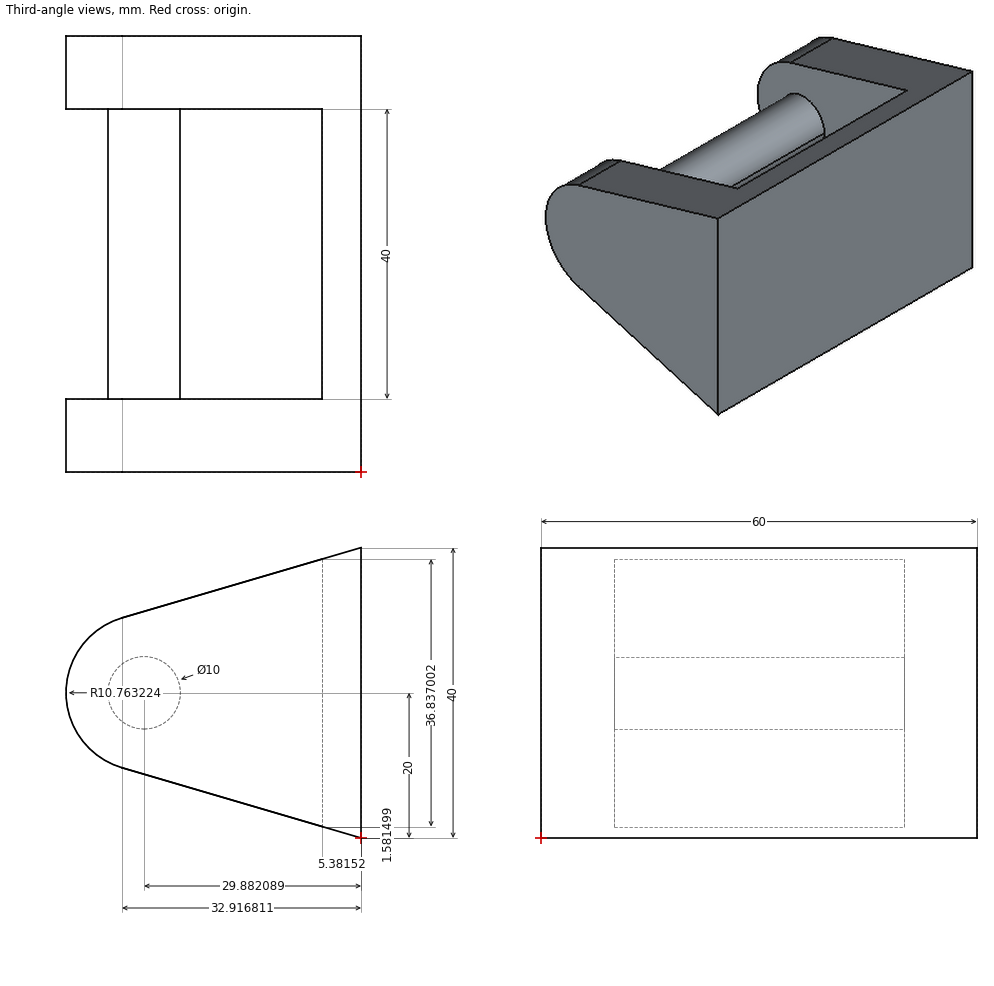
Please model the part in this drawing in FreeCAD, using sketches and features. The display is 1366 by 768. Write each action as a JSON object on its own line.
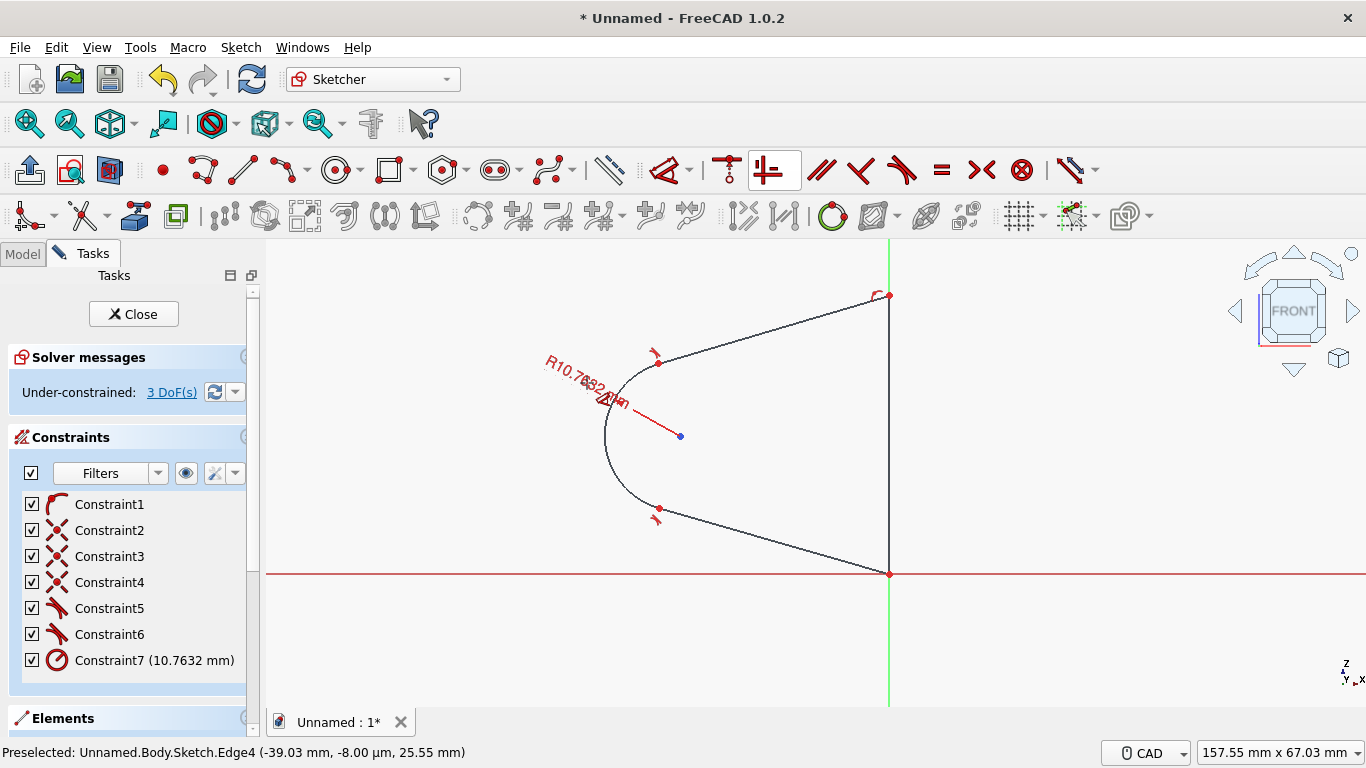
{"action": "left_click", "coordinate": [889, 379]}
{"action": "left_click", "coordinate": [923, 435]}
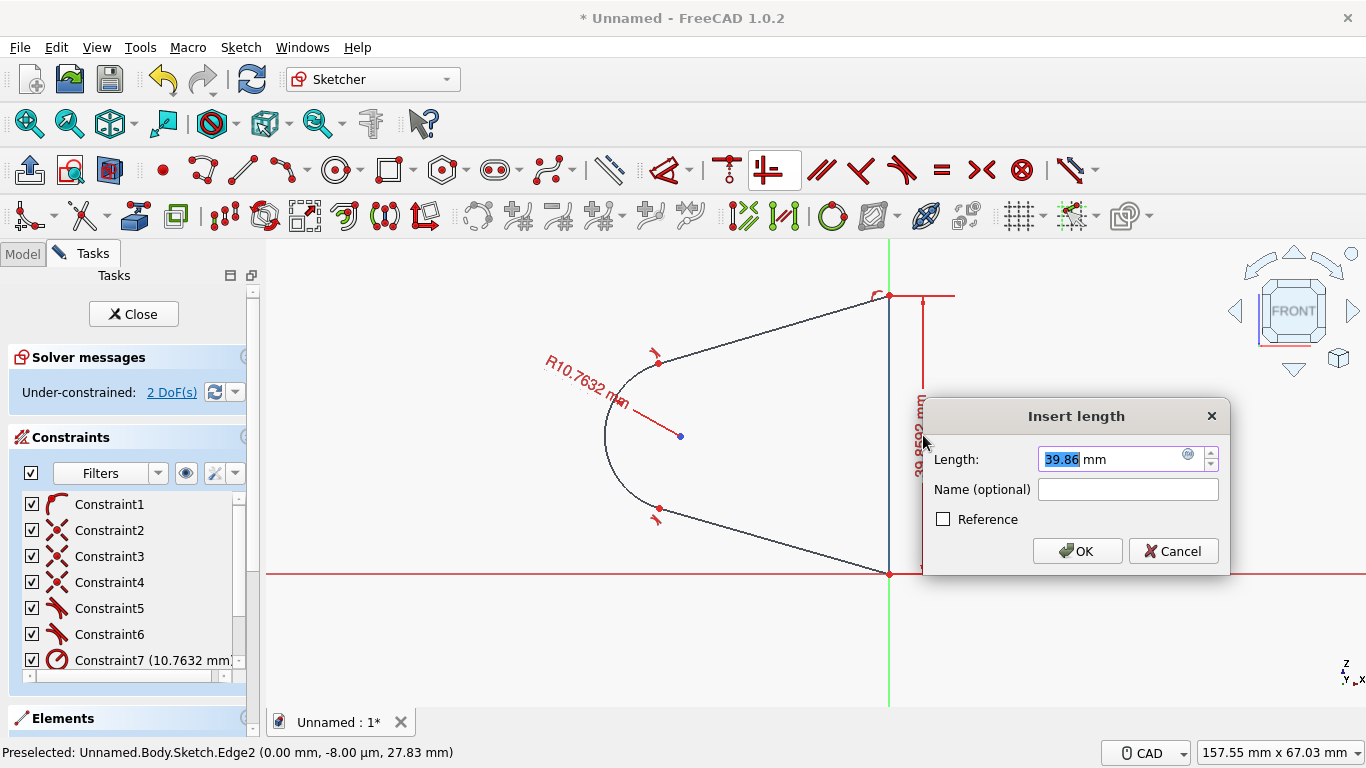
{"action": "type", "text": "40"}
{"action": "key", "text": "Return"}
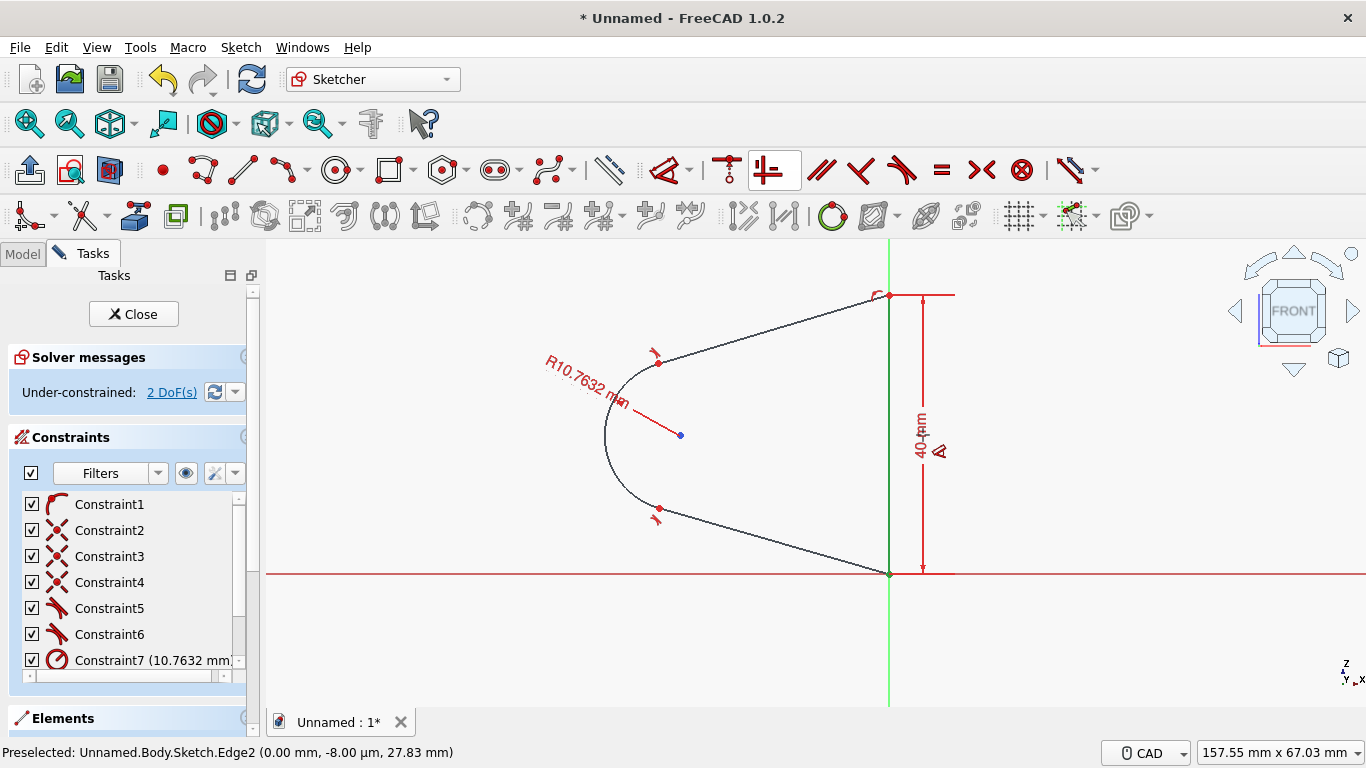
{"action": "left_click", "coordinate": [680, 436]}
{"action": "left_click", "coordinate": [923, 505]}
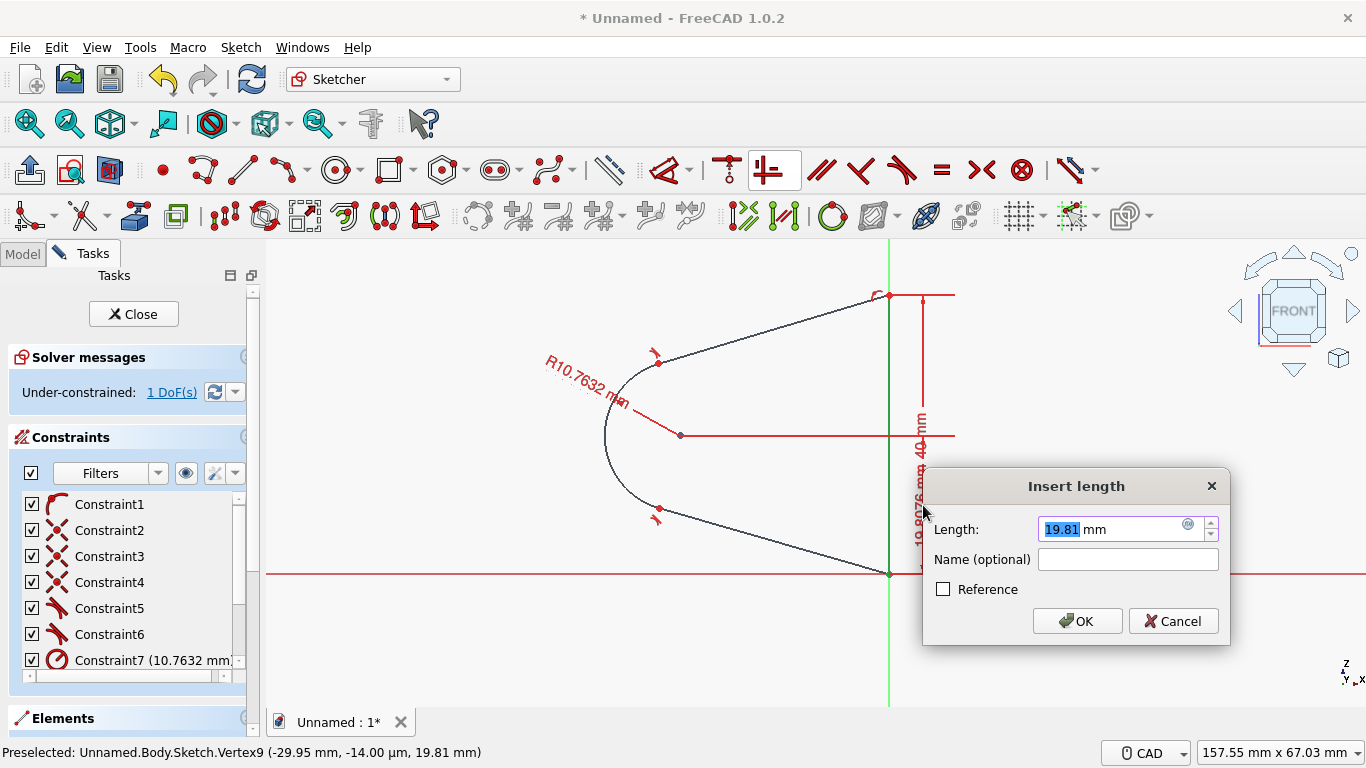
{"action": "type", "text": "20"}
{"action": "key", "text": "Return"}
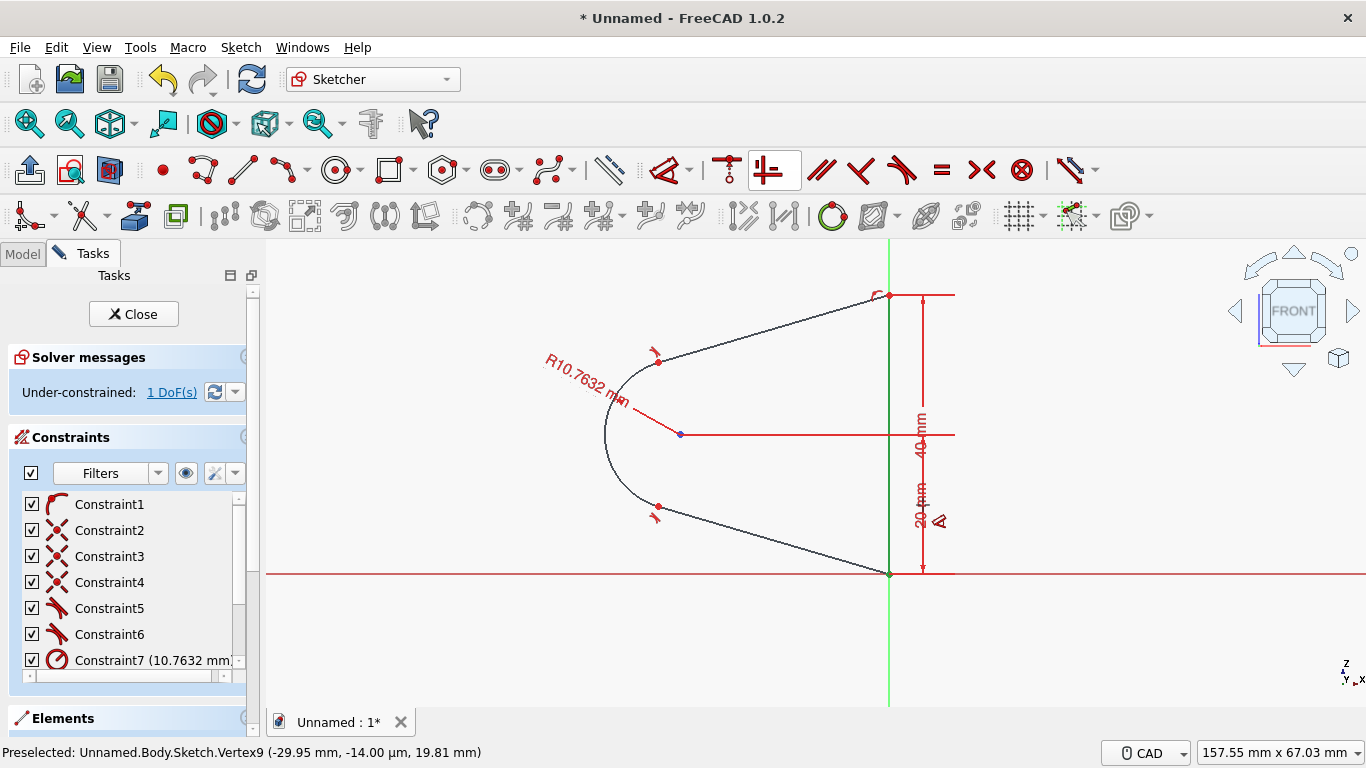
{"action": "left_click", "coordinate": [659, 363]}
{"action": "left_click", "coordinate": [774, 608]}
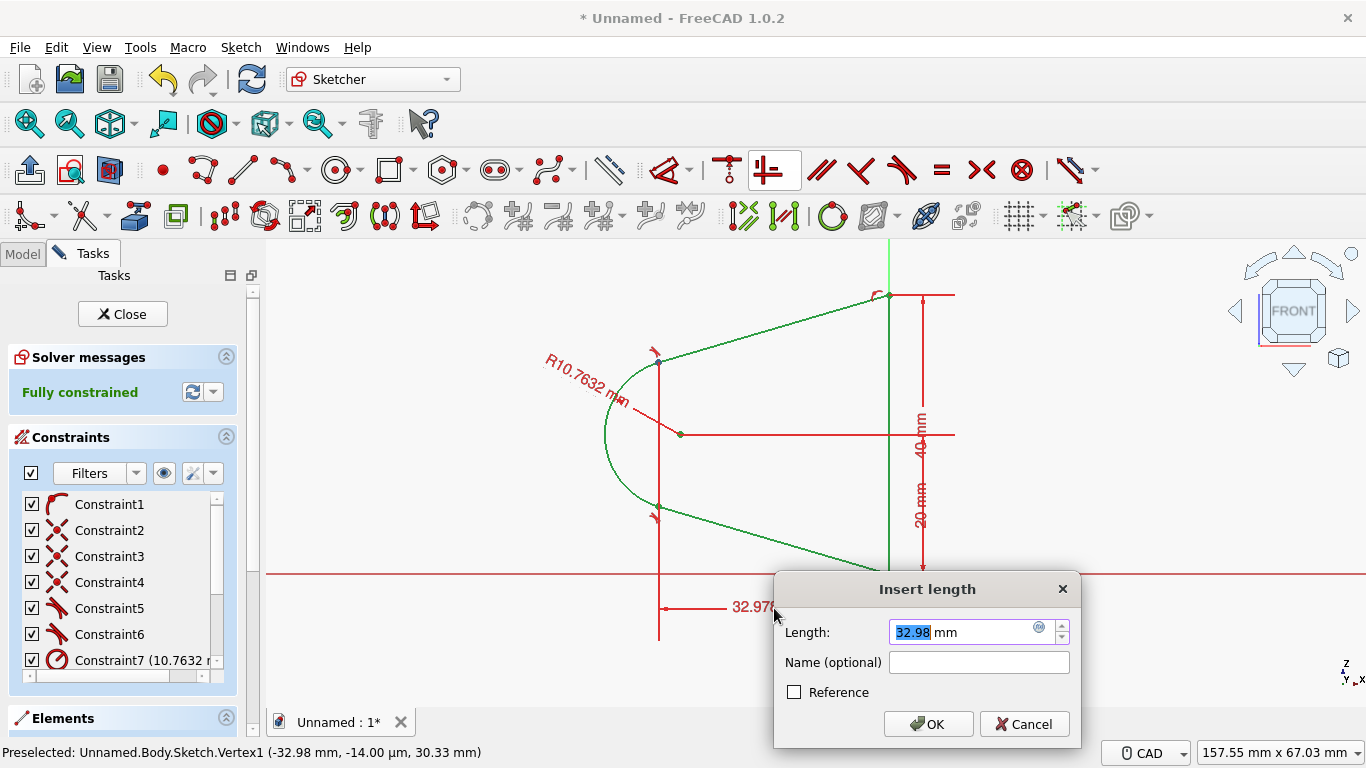
{"action": "type", "text": "32.916811"}
{"action": "key", "text": "Return"}
{"action": "key", "text": "Escape"}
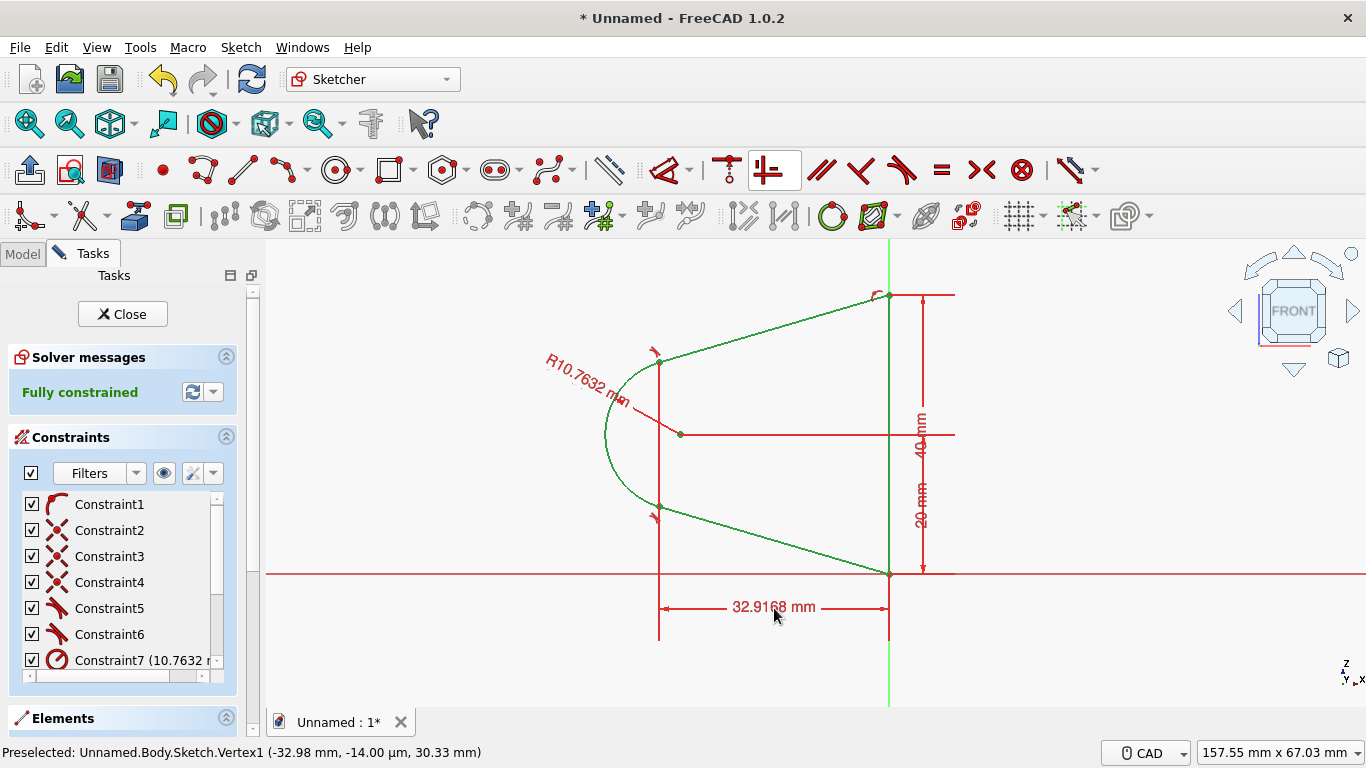
{"action": "left_click", "coordinate": [123, 314]}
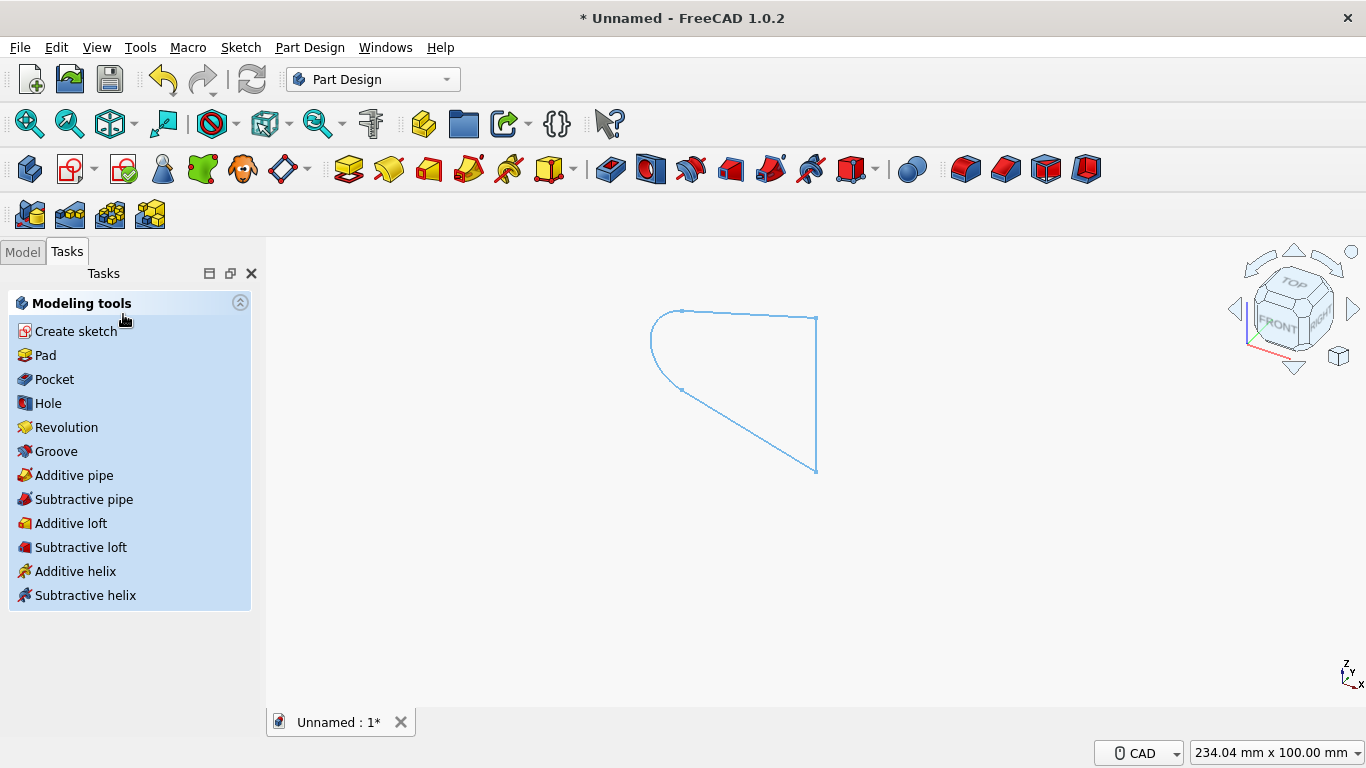
{"action": "left_click", "coordinate": [350, 170]}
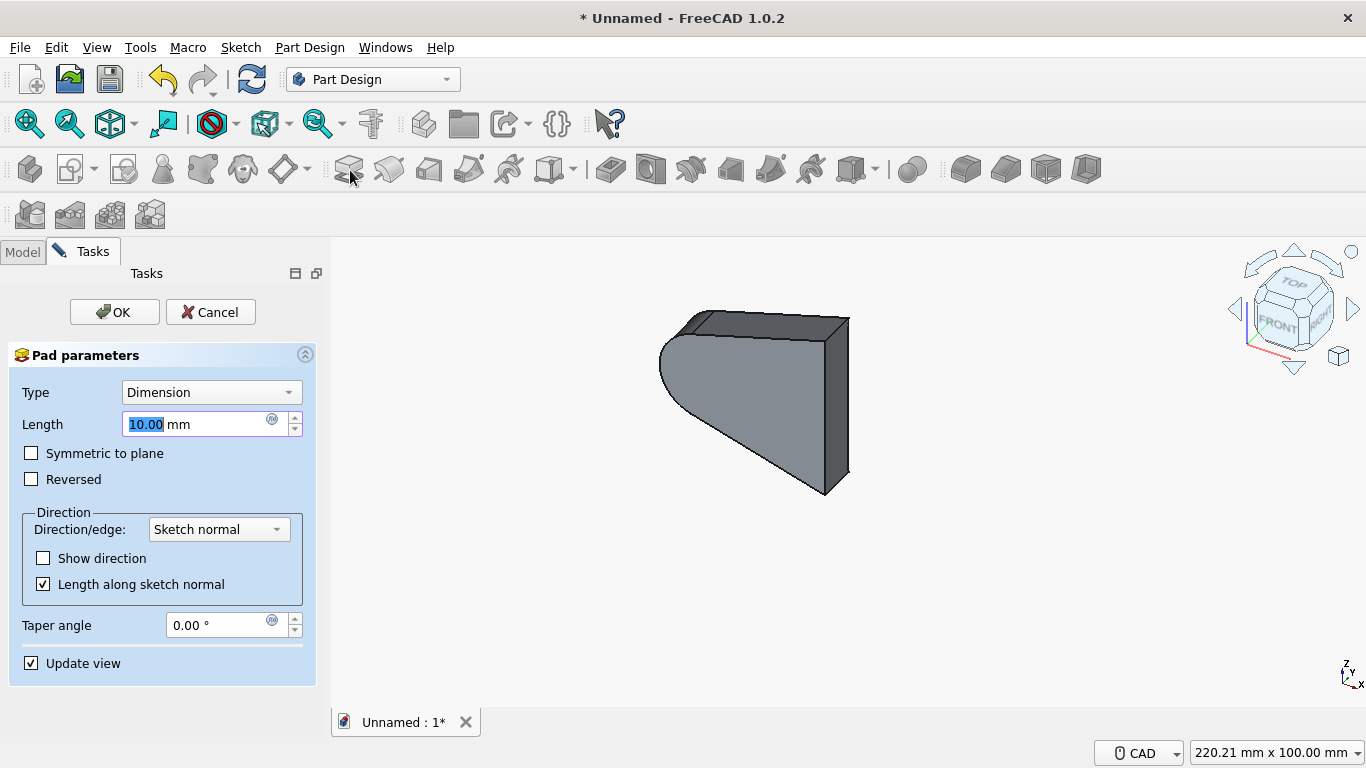
{"action": "type", "text": "60"}
{"action": "key", "text": "Tab"}